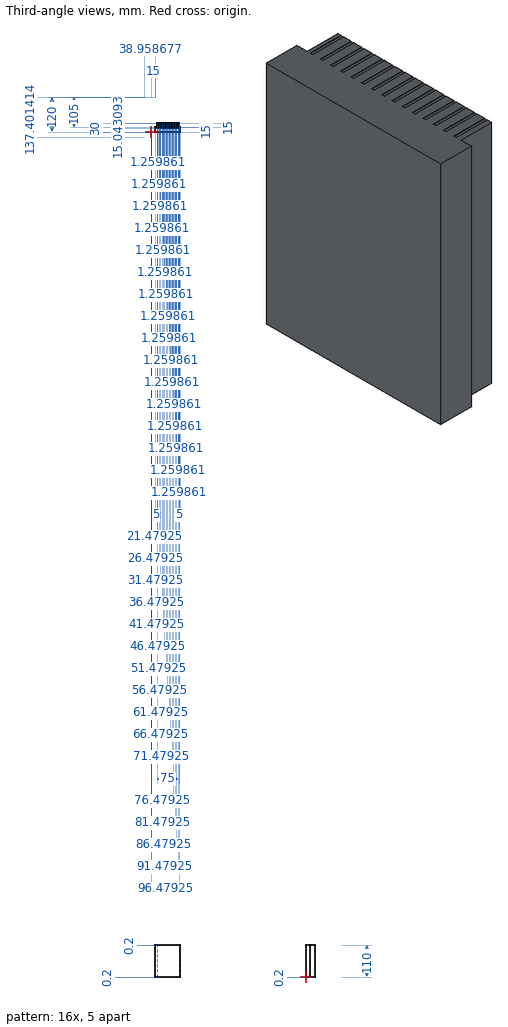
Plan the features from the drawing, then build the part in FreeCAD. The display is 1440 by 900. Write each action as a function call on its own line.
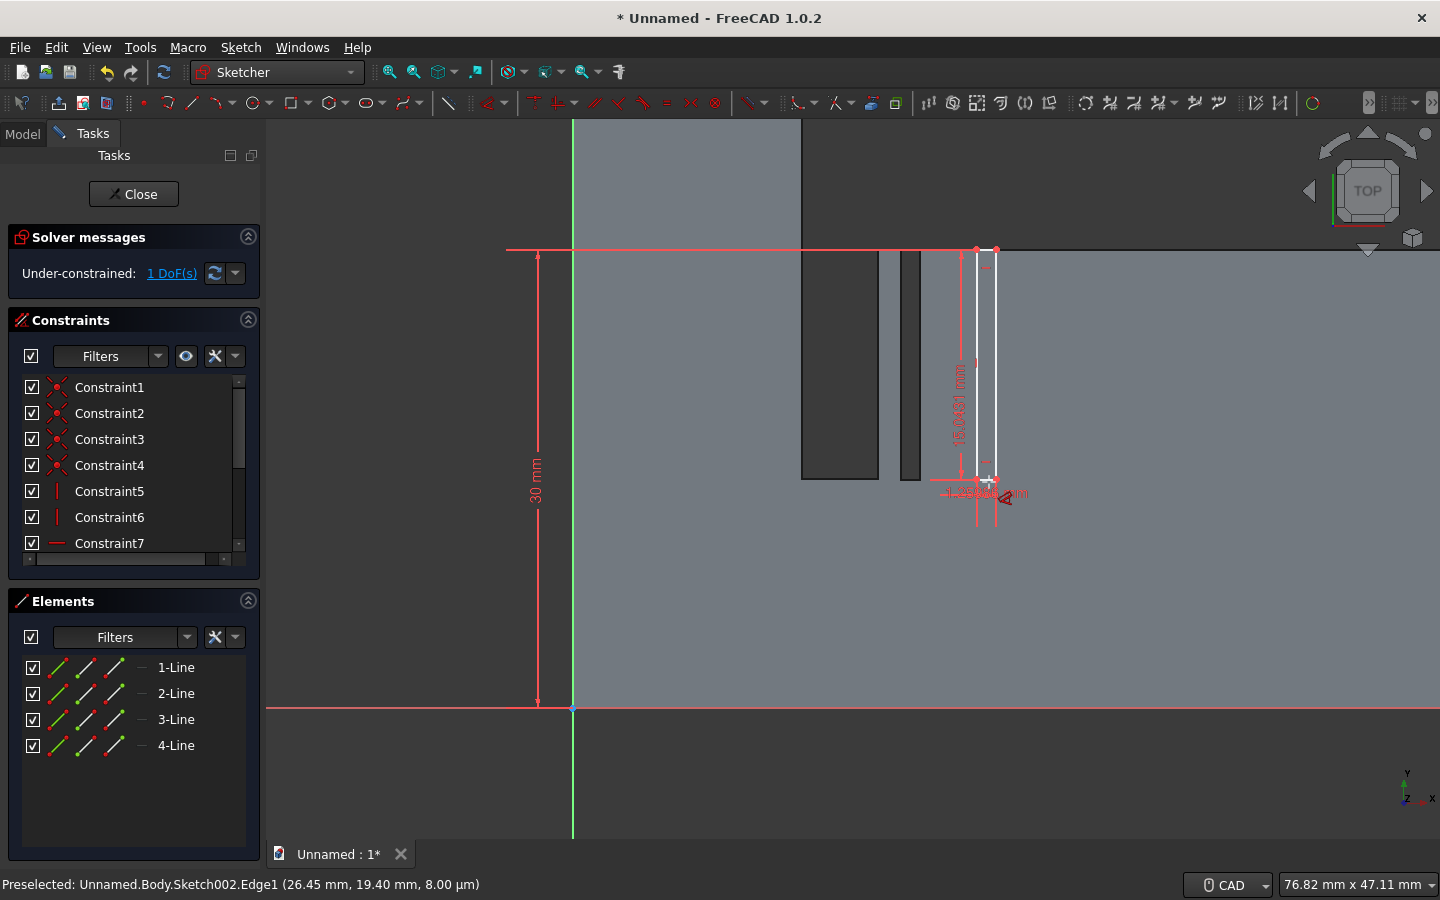
click(977, 250)
click(775, 742)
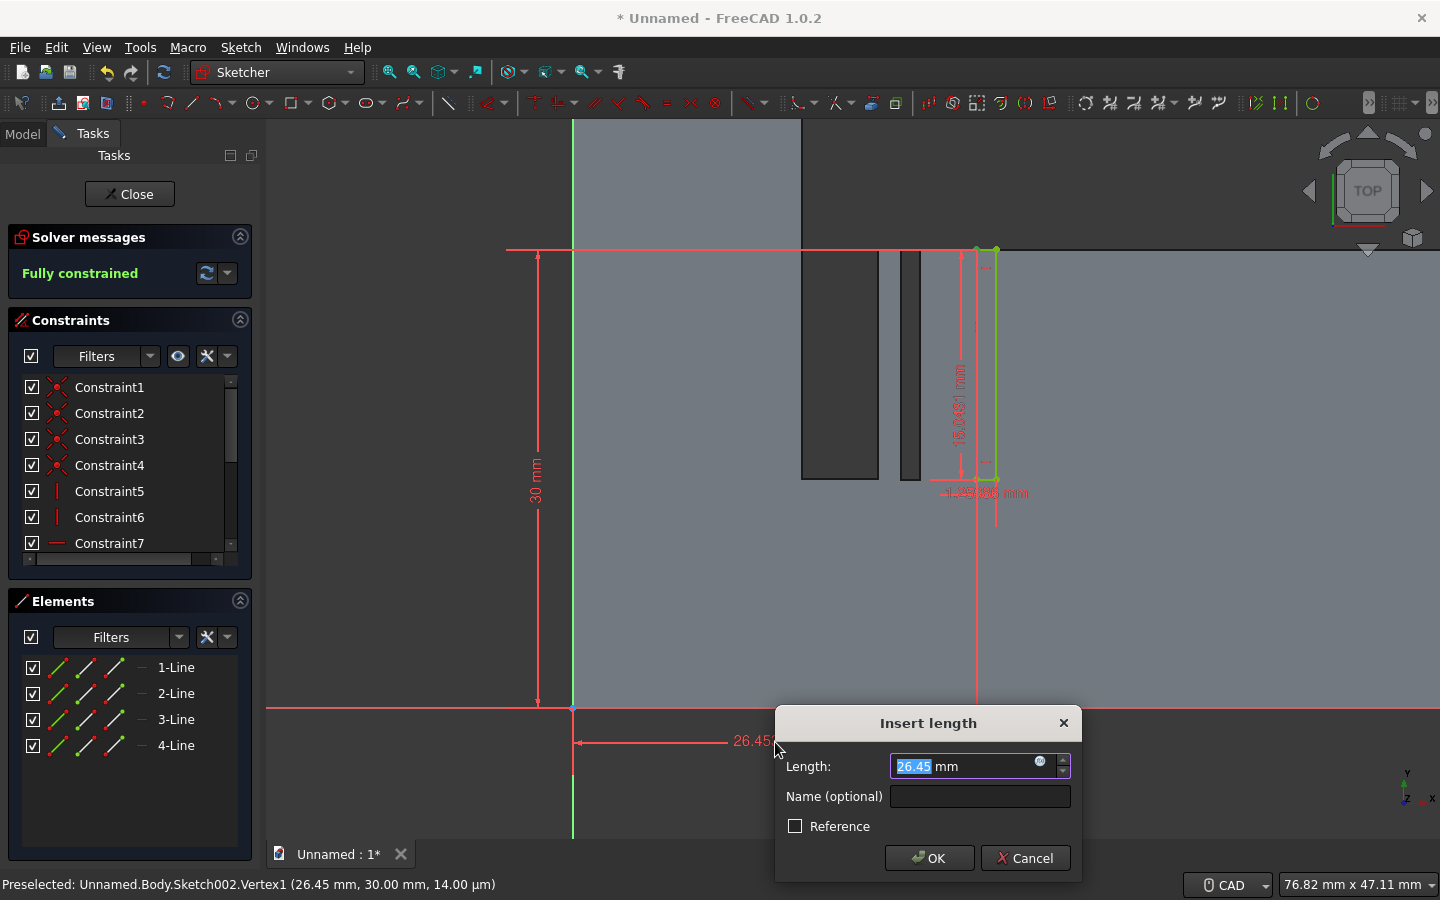
text(26.47925)
key(Return)
key(Escape)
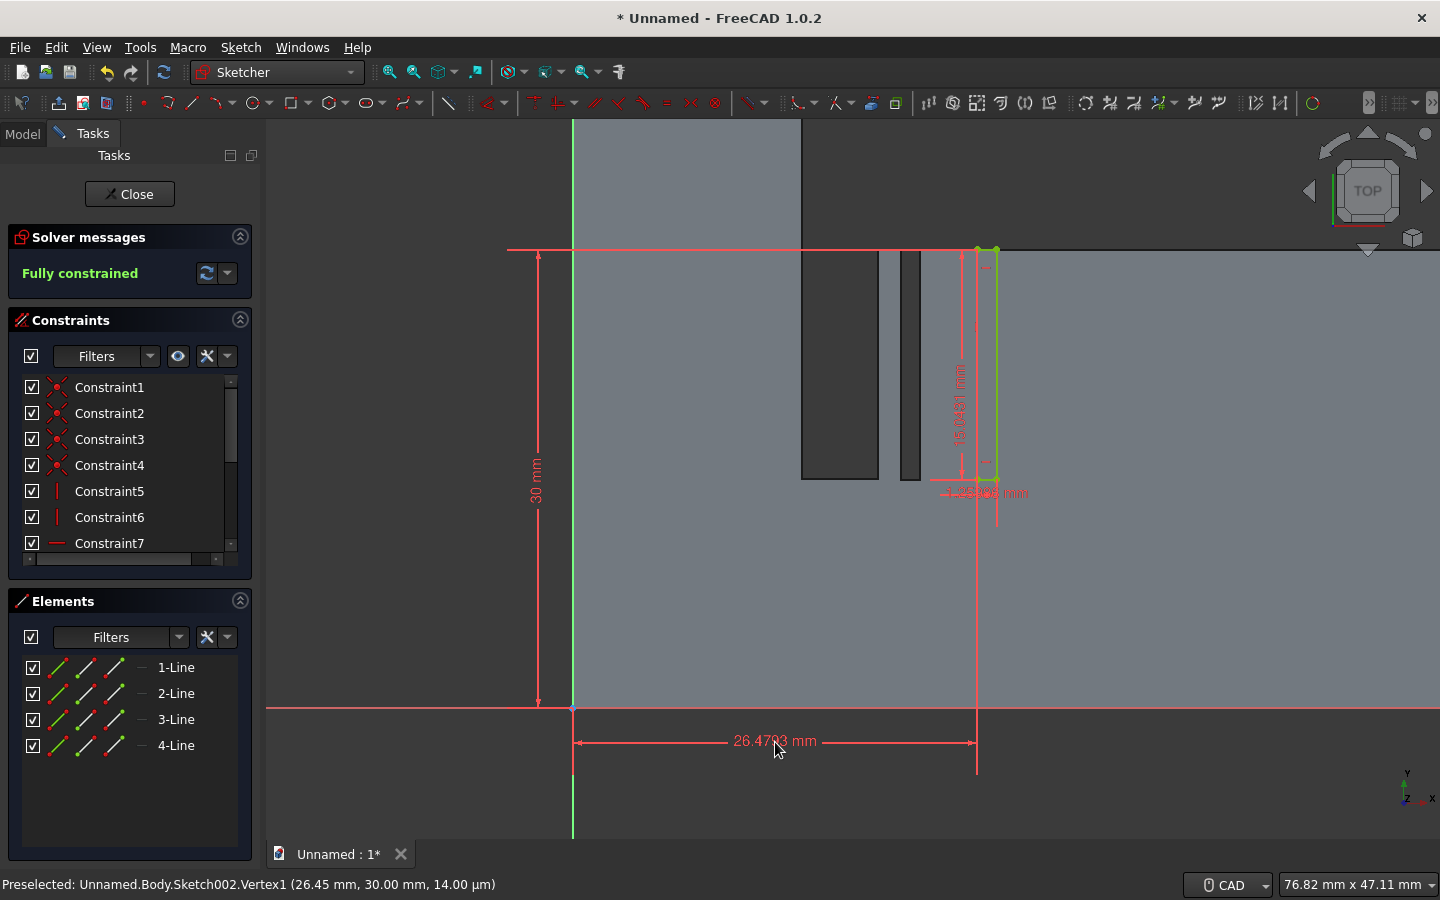
click(130, 194)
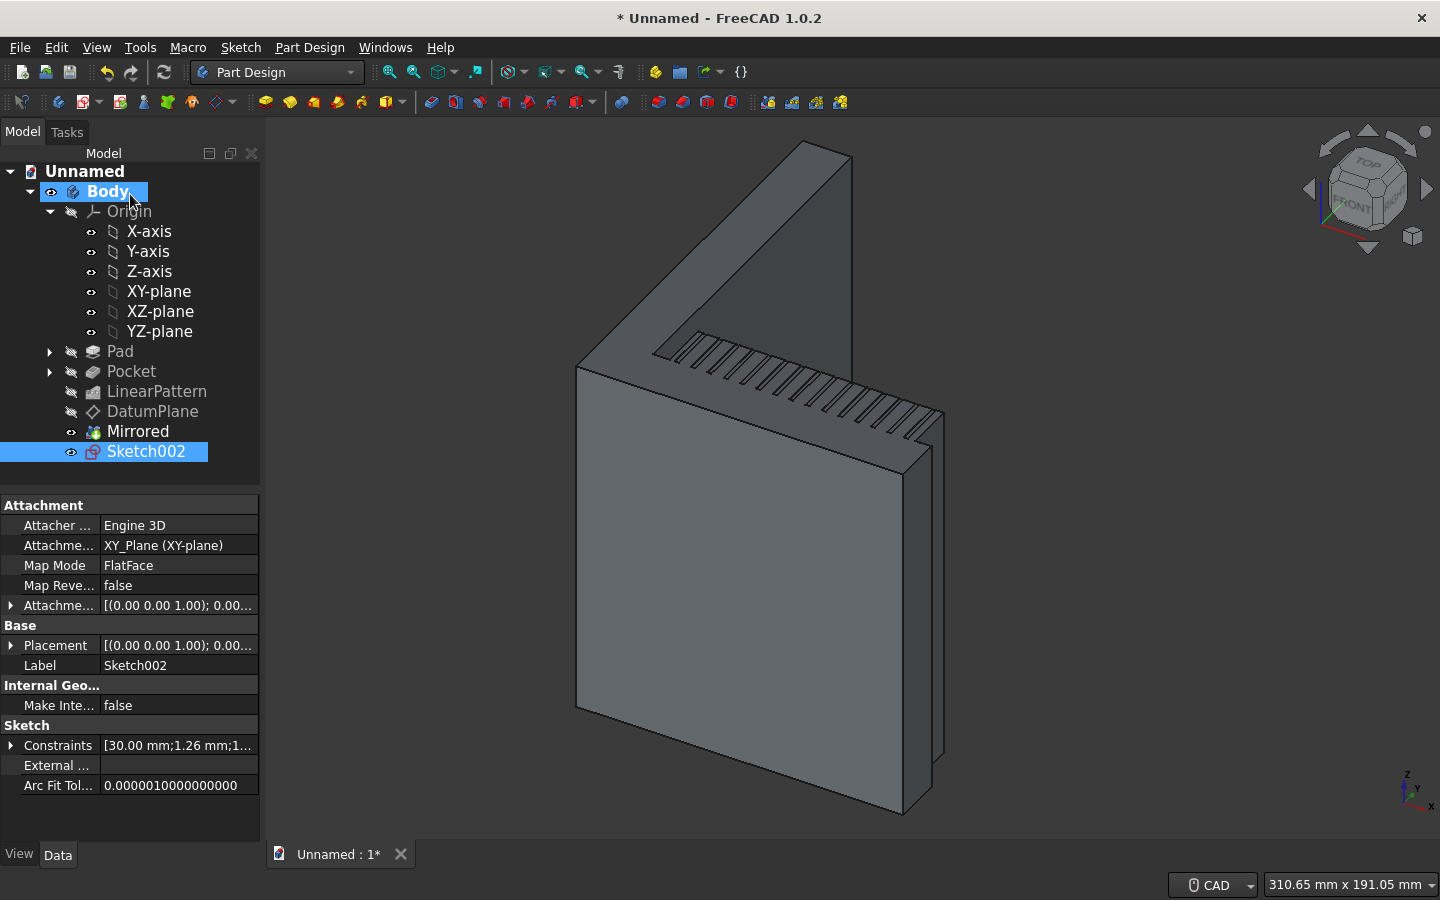
click(432, 102)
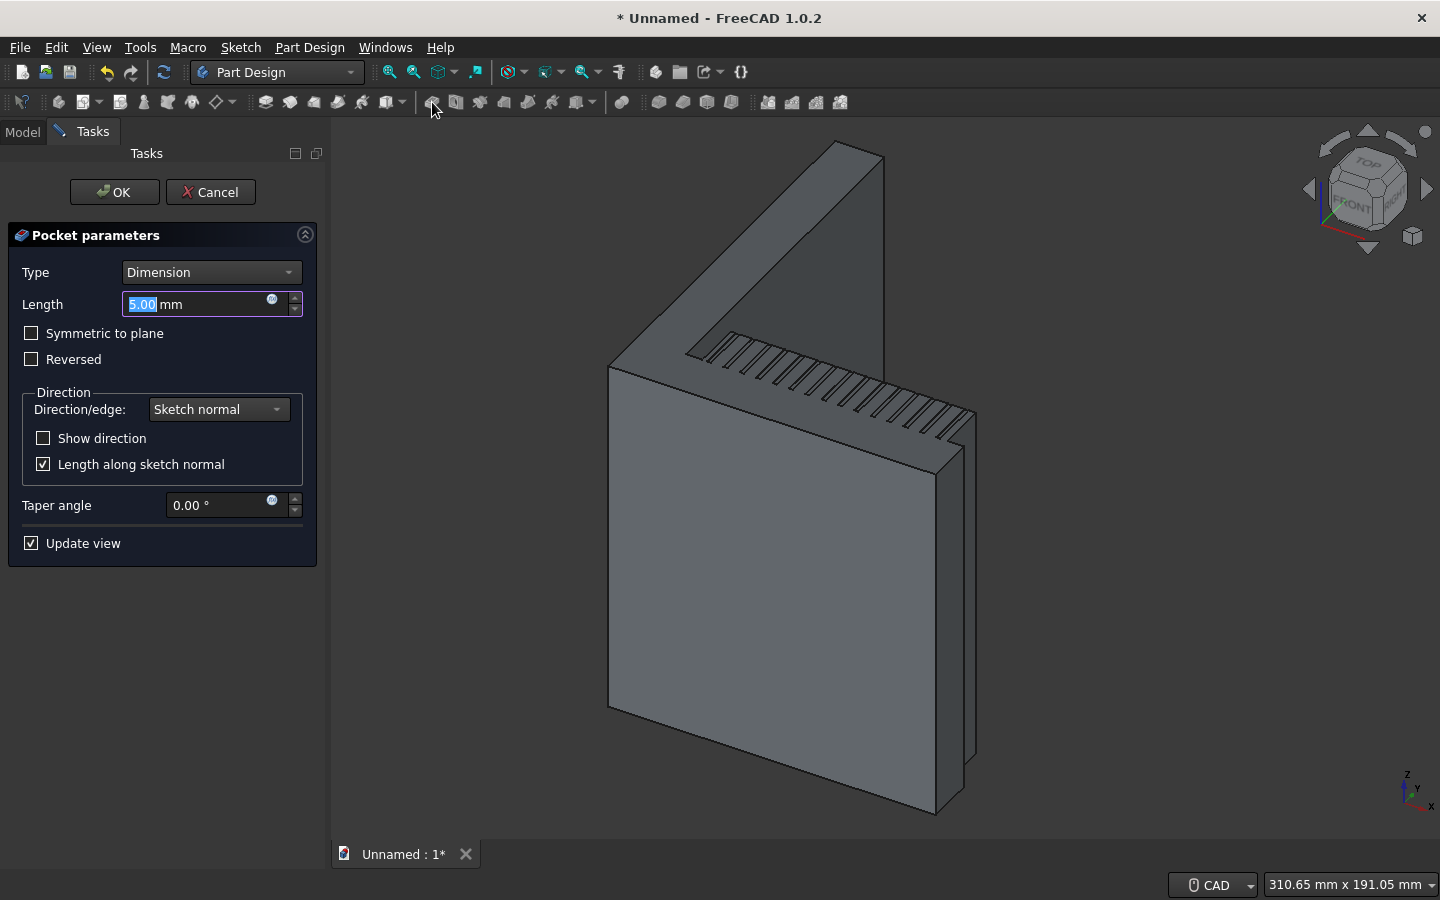
text(0.2)
key(Tab)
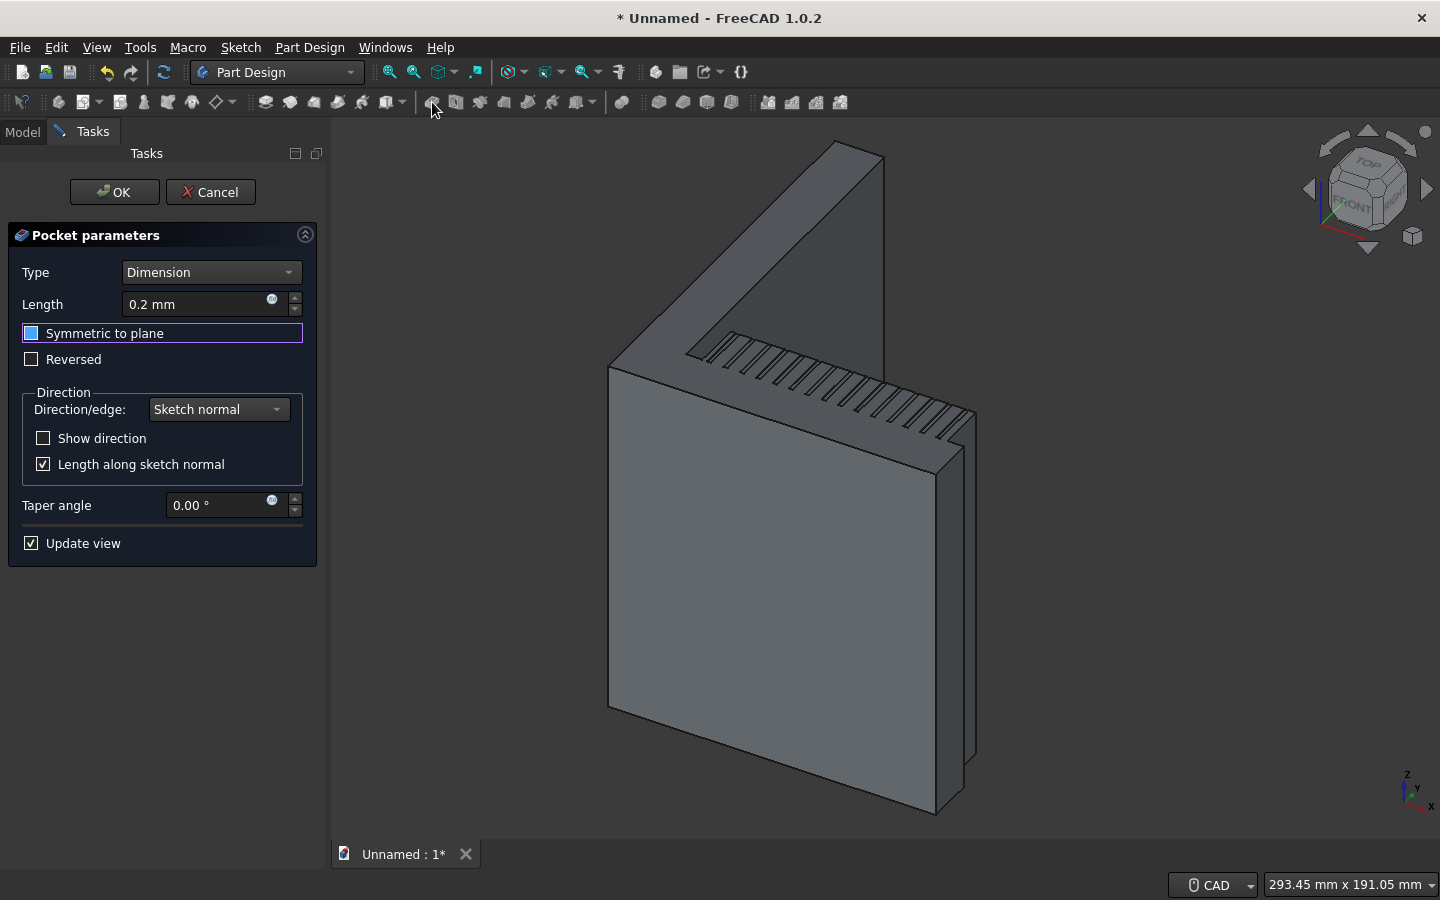
click(30, 359)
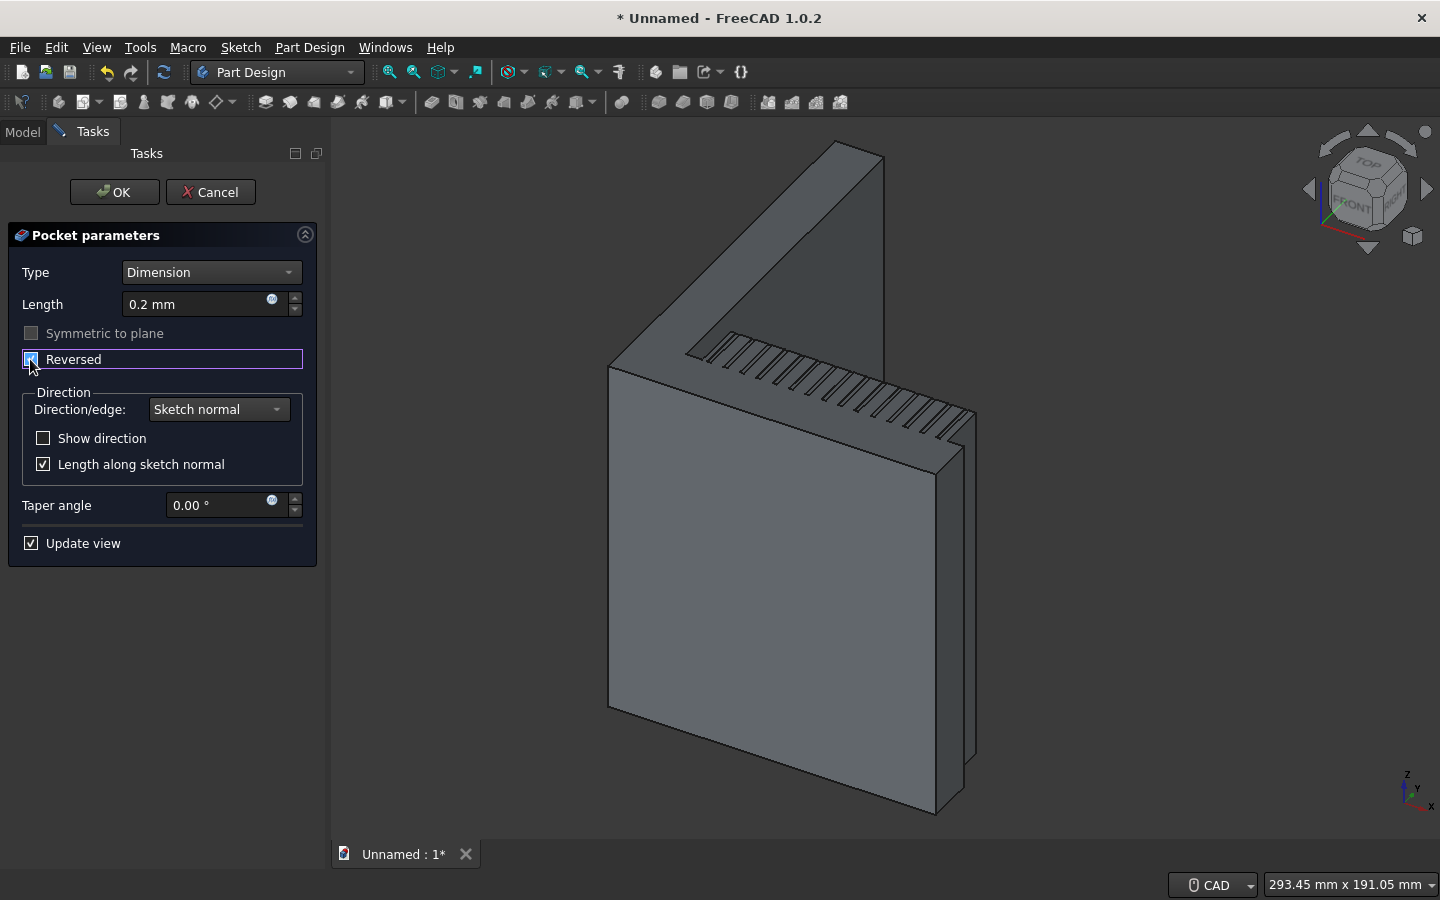
click(115, 192)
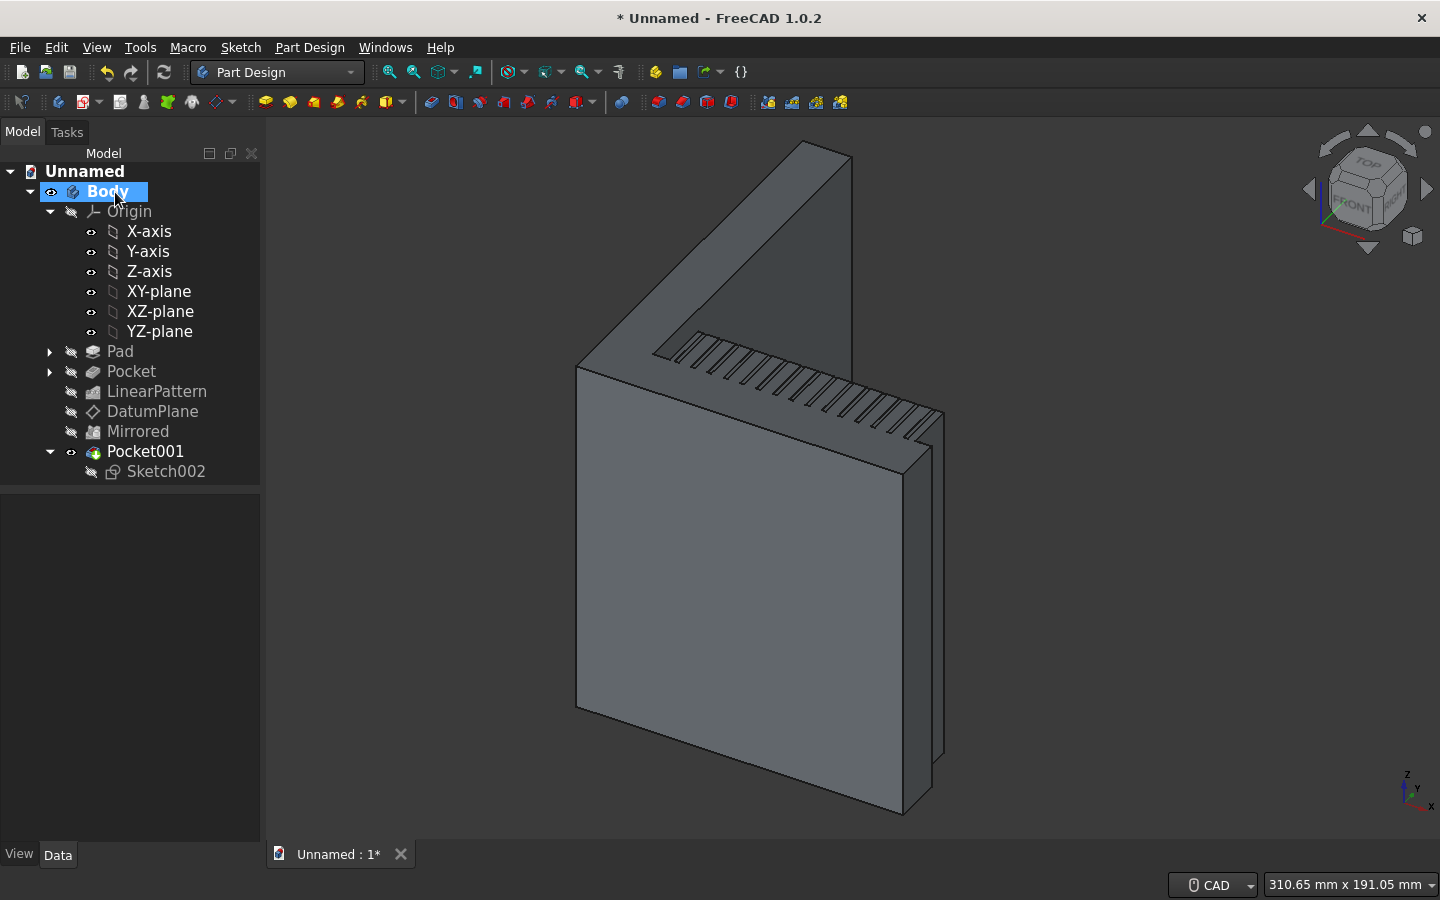
click(84, 102)